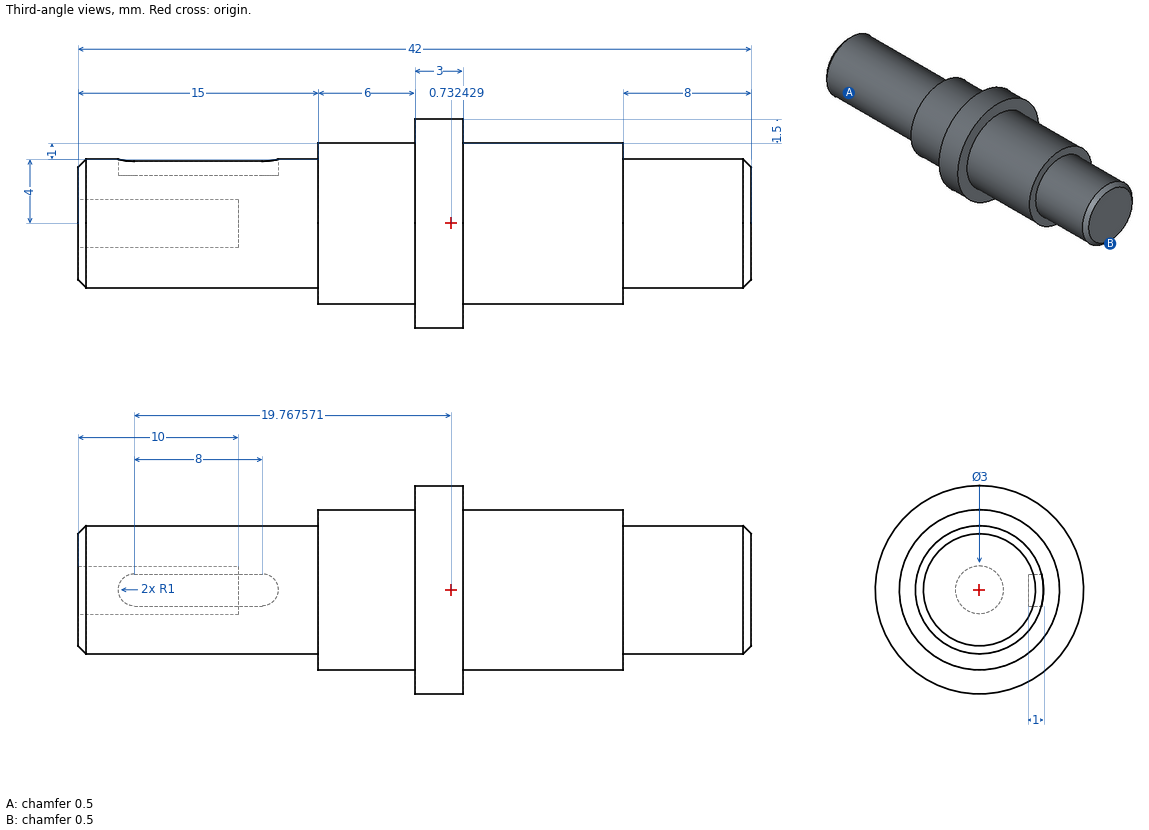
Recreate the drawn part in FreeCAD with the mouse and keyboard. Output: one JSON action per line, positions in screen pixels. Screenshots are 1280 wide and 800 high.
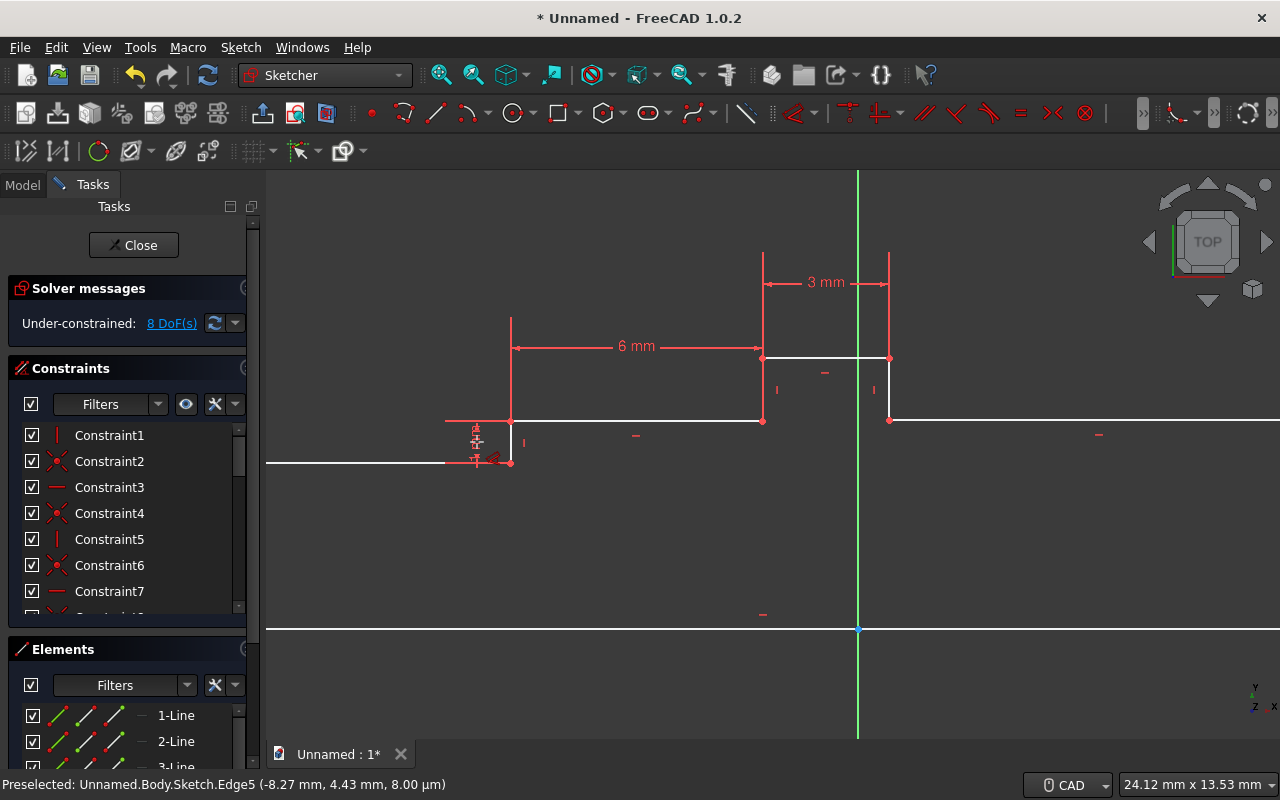
{"action": "scroll", "coordinate": [679, 438], "scroll_direction": "down", "scroll_amount": 6}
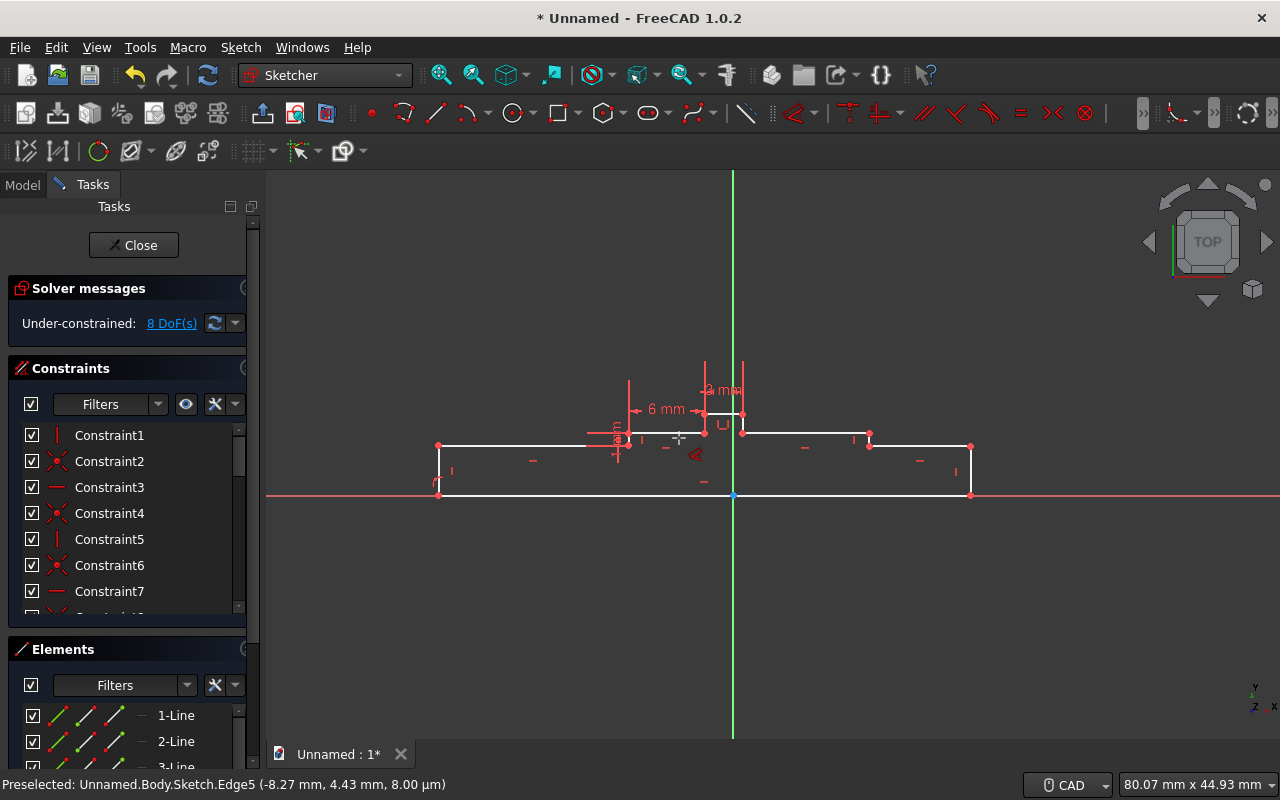
{"action": "left_click", "coordinate": [439, 461]}
{"action": "left_click", "coordinate": [405, 471]}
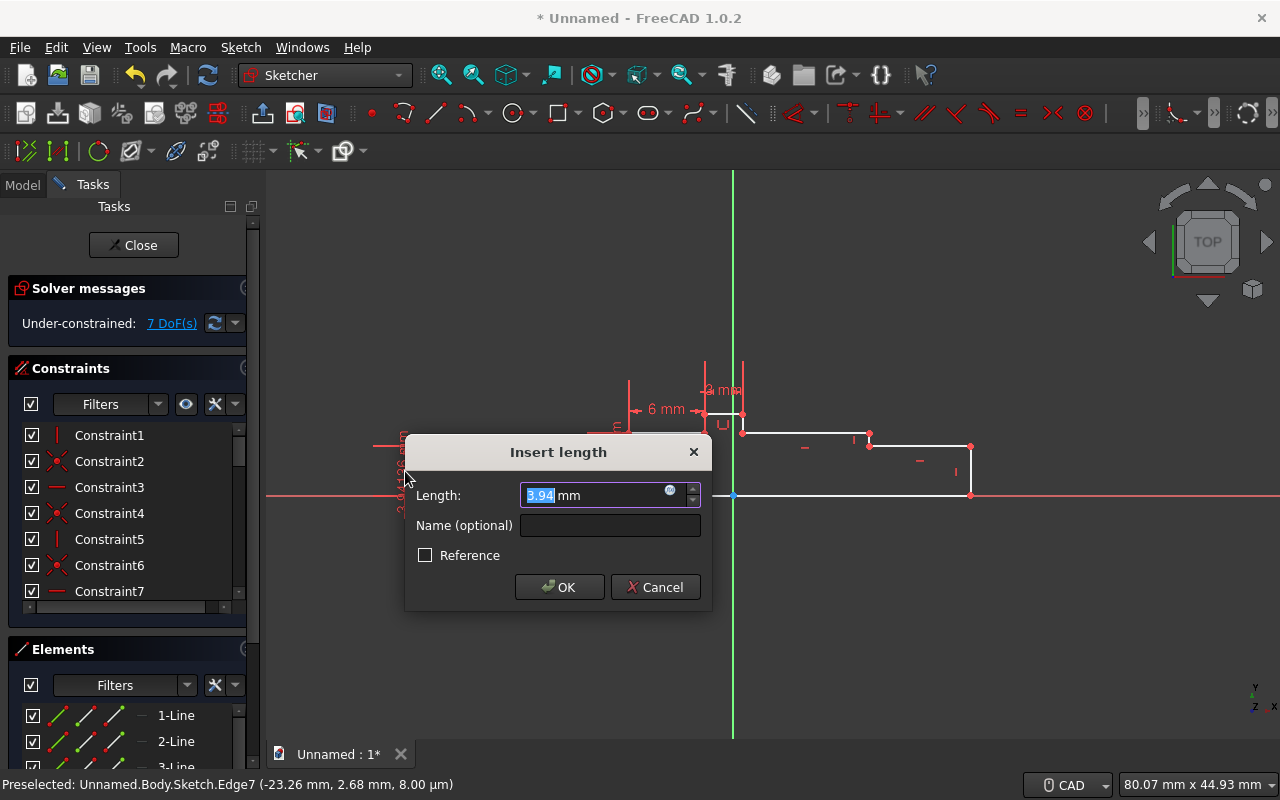
{"action": "type", "text": "4"}
{"action": "key", "text": "Return"}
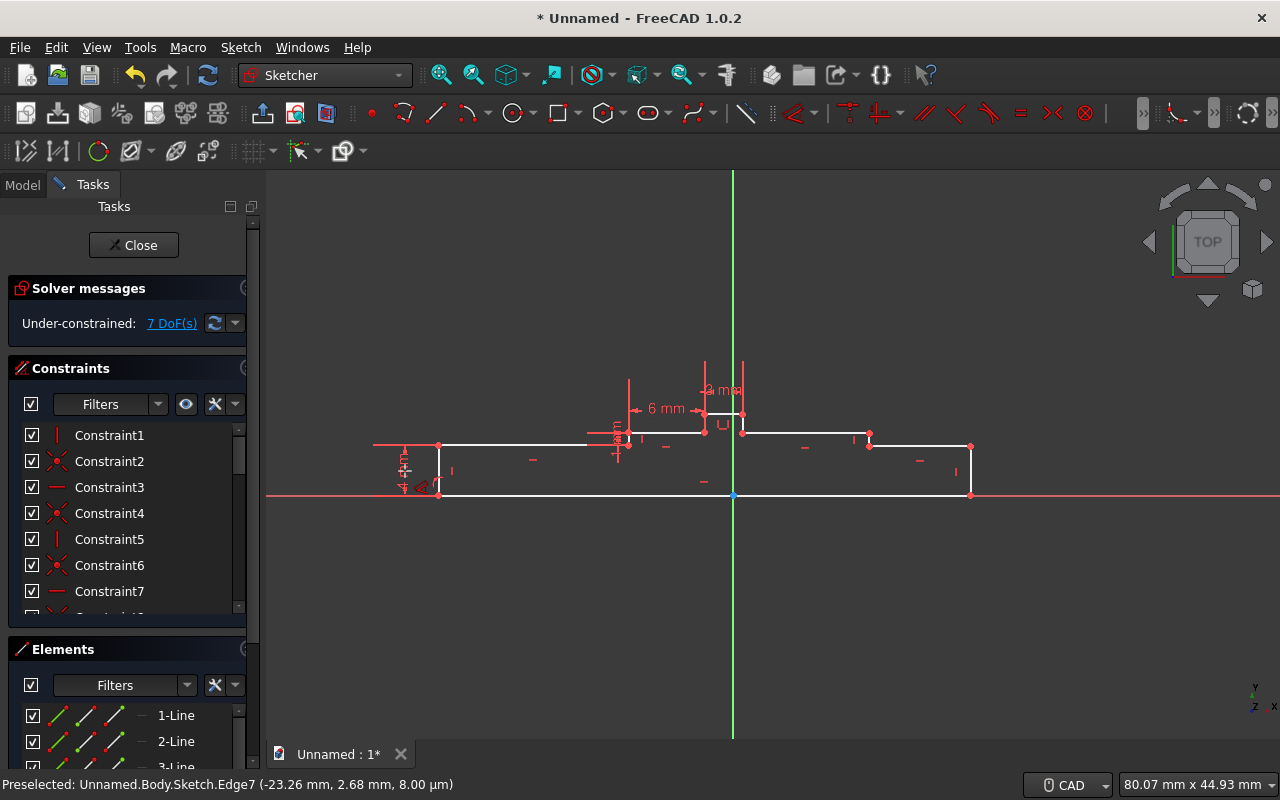
{"action": "left_click", "coordinate": [971, 481]}
{"action": "left_click", "coordinate": [1005, 471]}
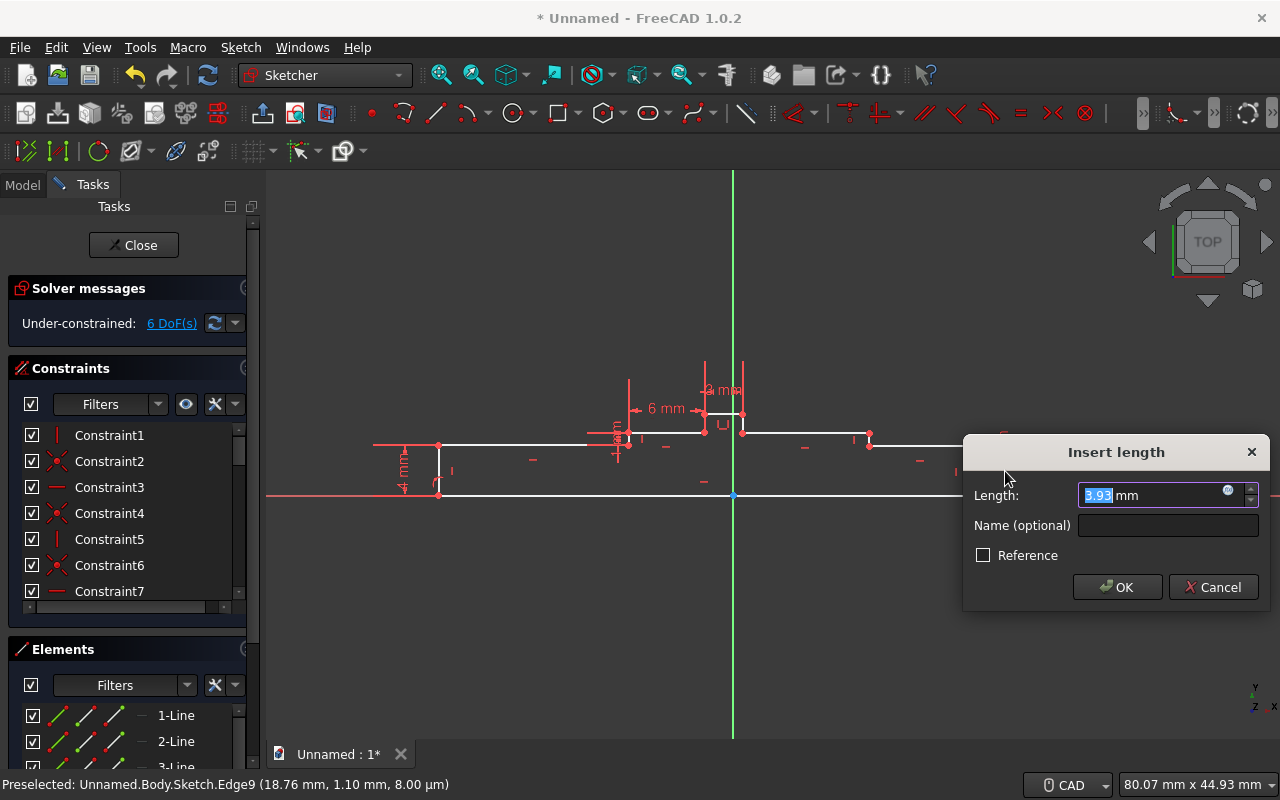
{"action": "type", "text": "4"}
{"action": "key", "text": "Return"}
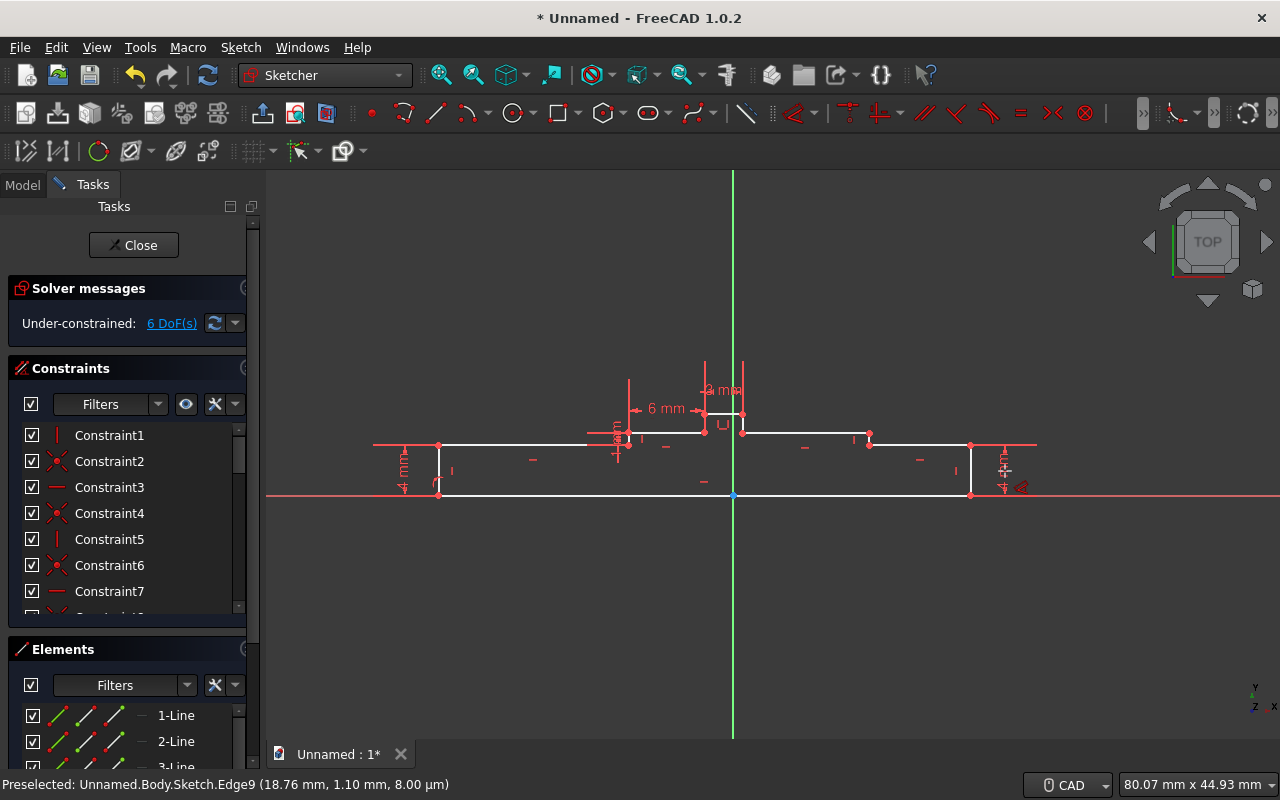
{"action": "left_click", "coordinate": [940, 445]}
{"action": "left_click", "coordinate": [920, 411]}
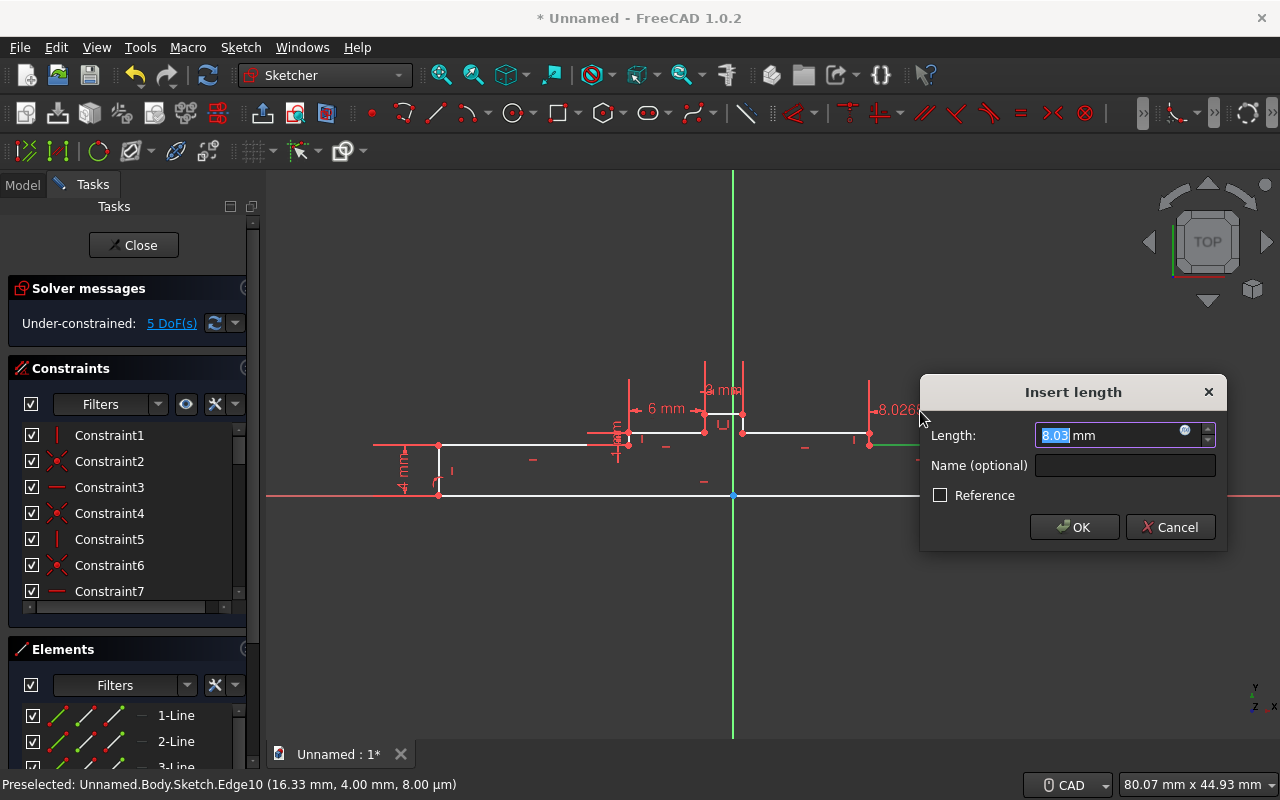
{"action": "type", "text": "8"}
{"action": "key", "text": "Return"}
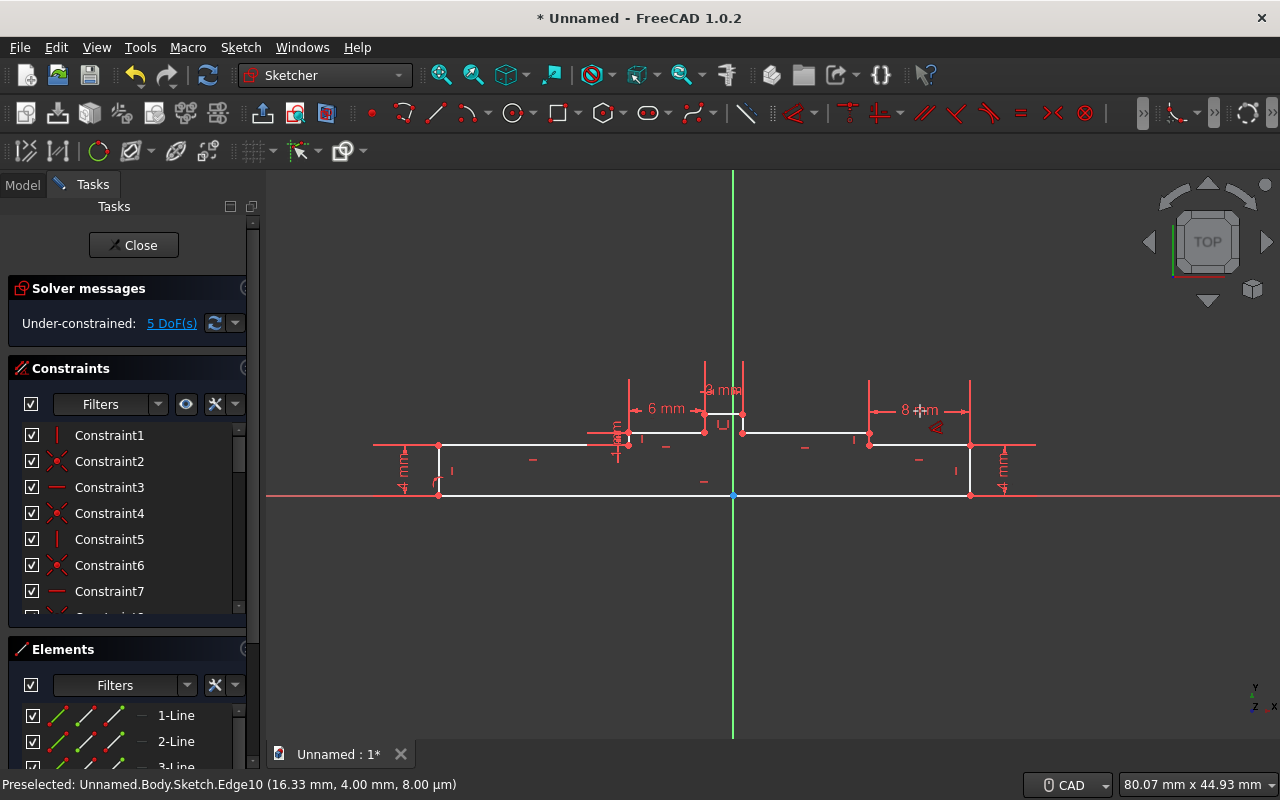
{"action": "scroll", "coordinate": [869, 439], "scroll_direction": "up", "scroll_amount": 6}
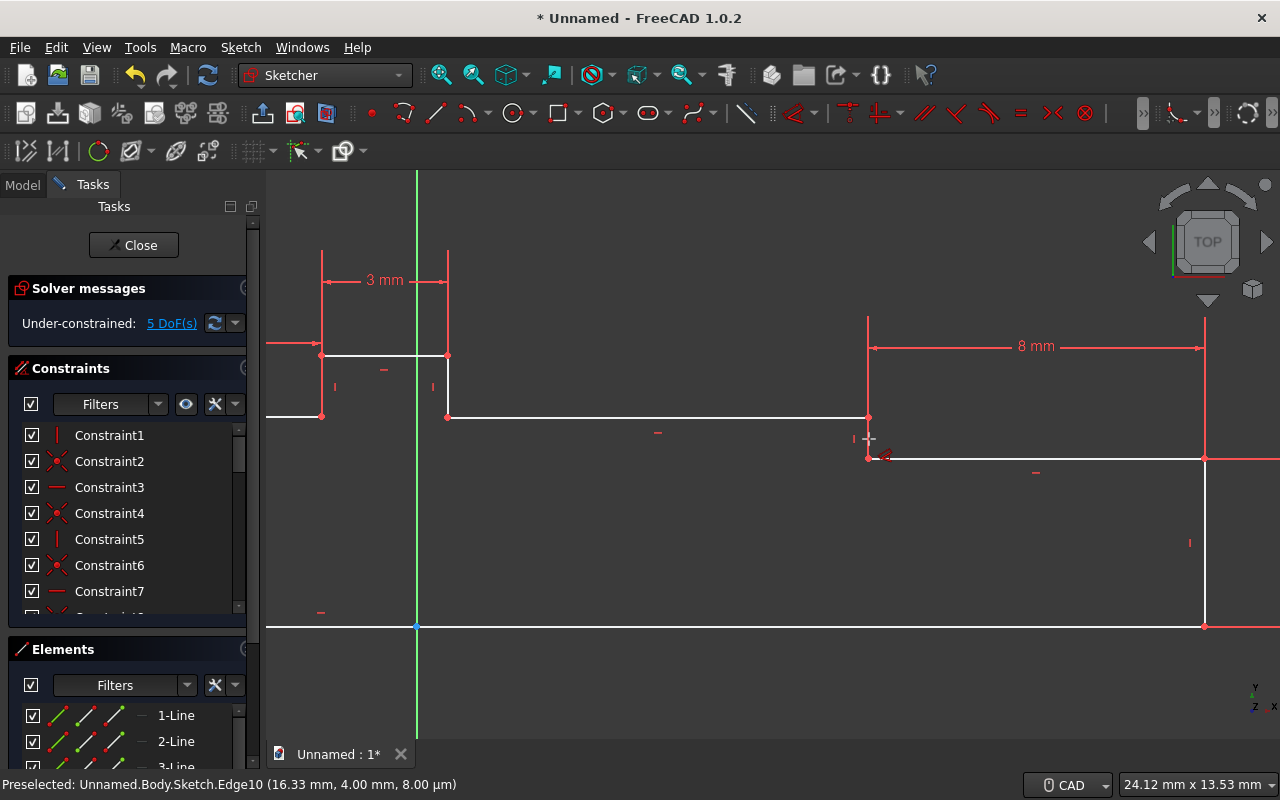
{"action": "left_click", "coordinate": [868, 438]}
{"action": "left_click", "coordinate": [902, 438]}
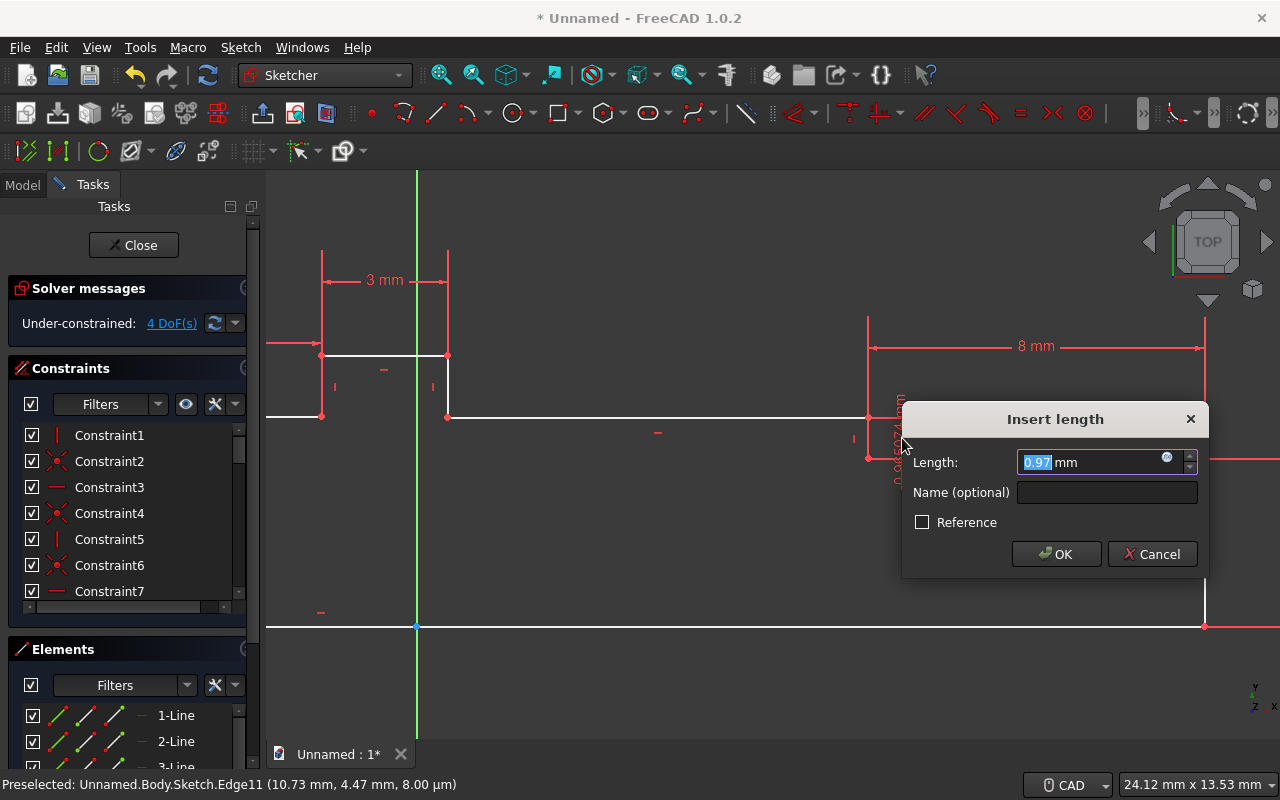
{"action": "type", "text": "1"}
{"action": "key", "text": "Return"}